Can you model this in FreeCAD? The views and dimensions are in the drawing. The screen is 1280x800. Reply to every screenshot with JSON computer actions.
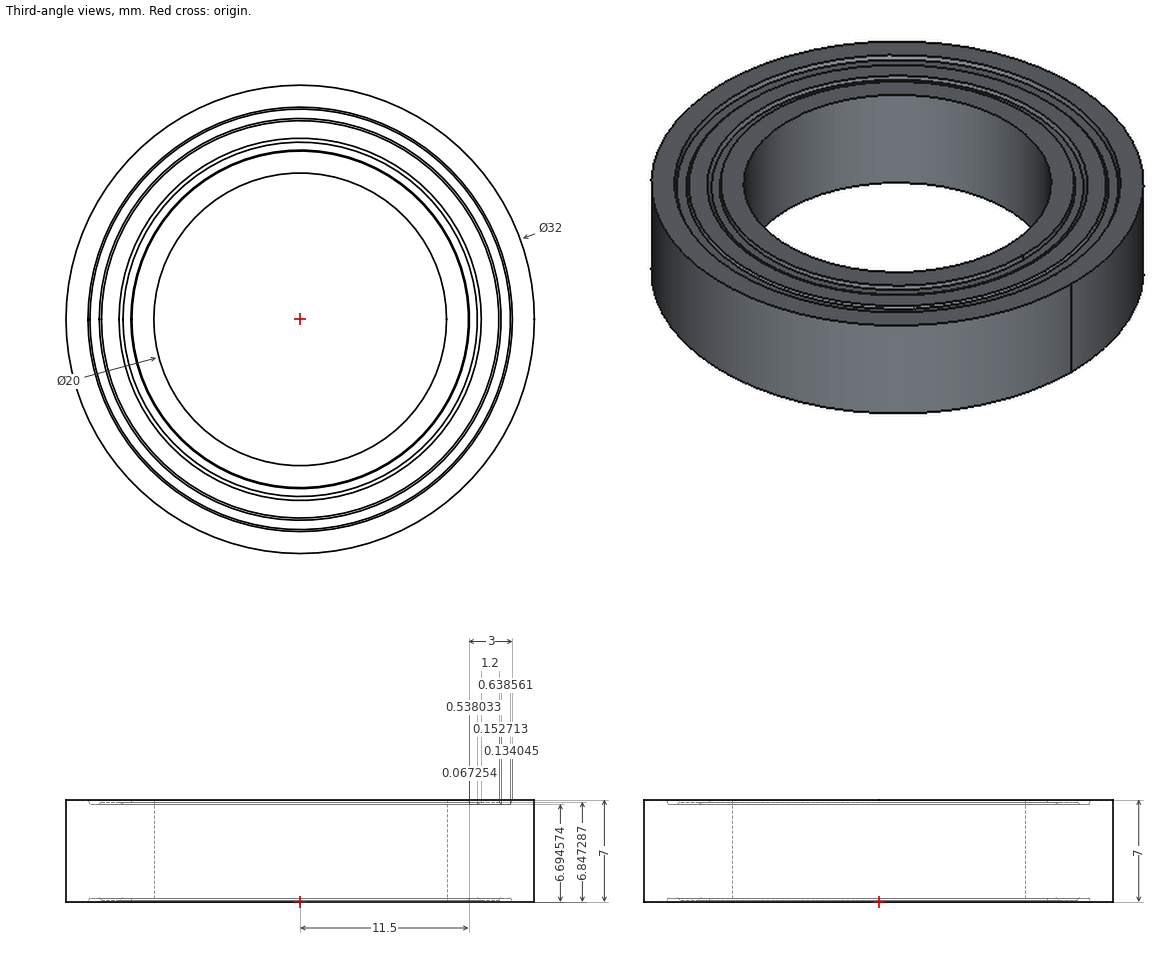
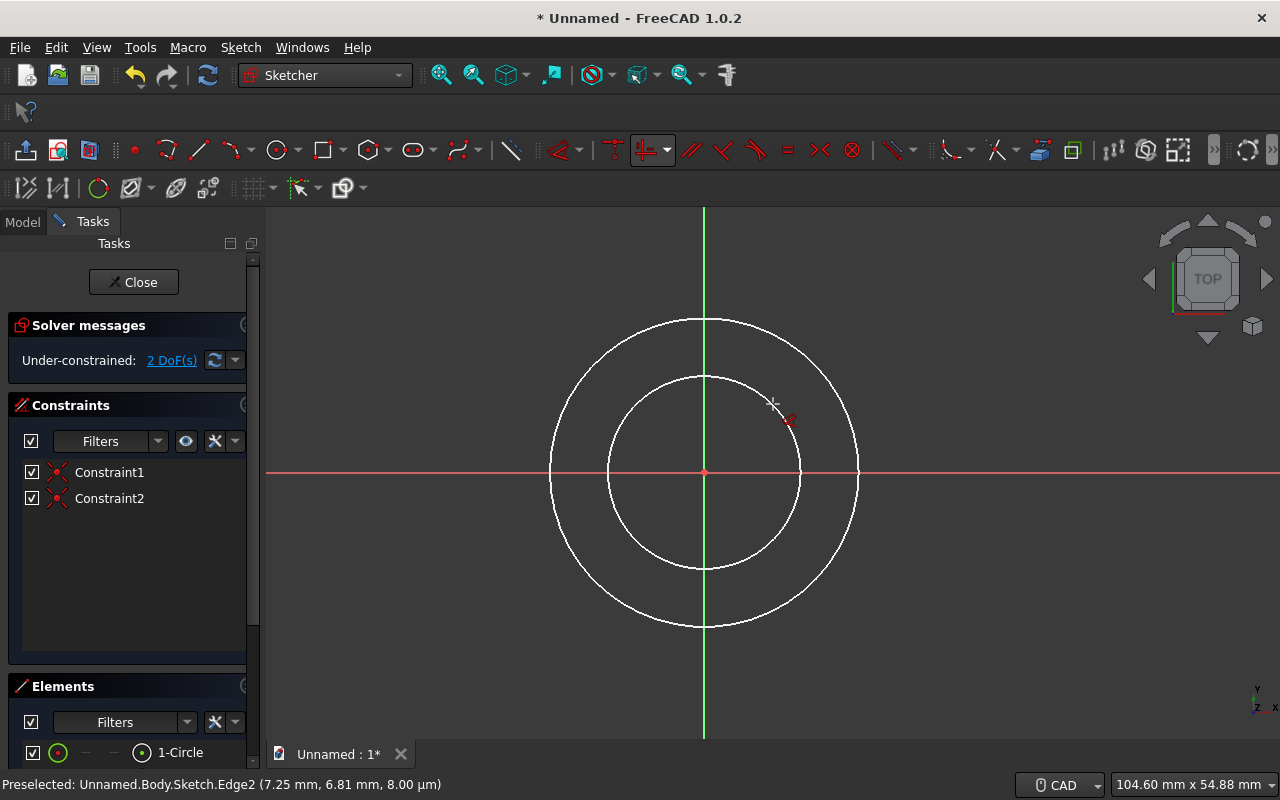
{"action": "left_click", "coordinate": [813, 363]}
{"action": "left_click", "coordinate": [836, 340]}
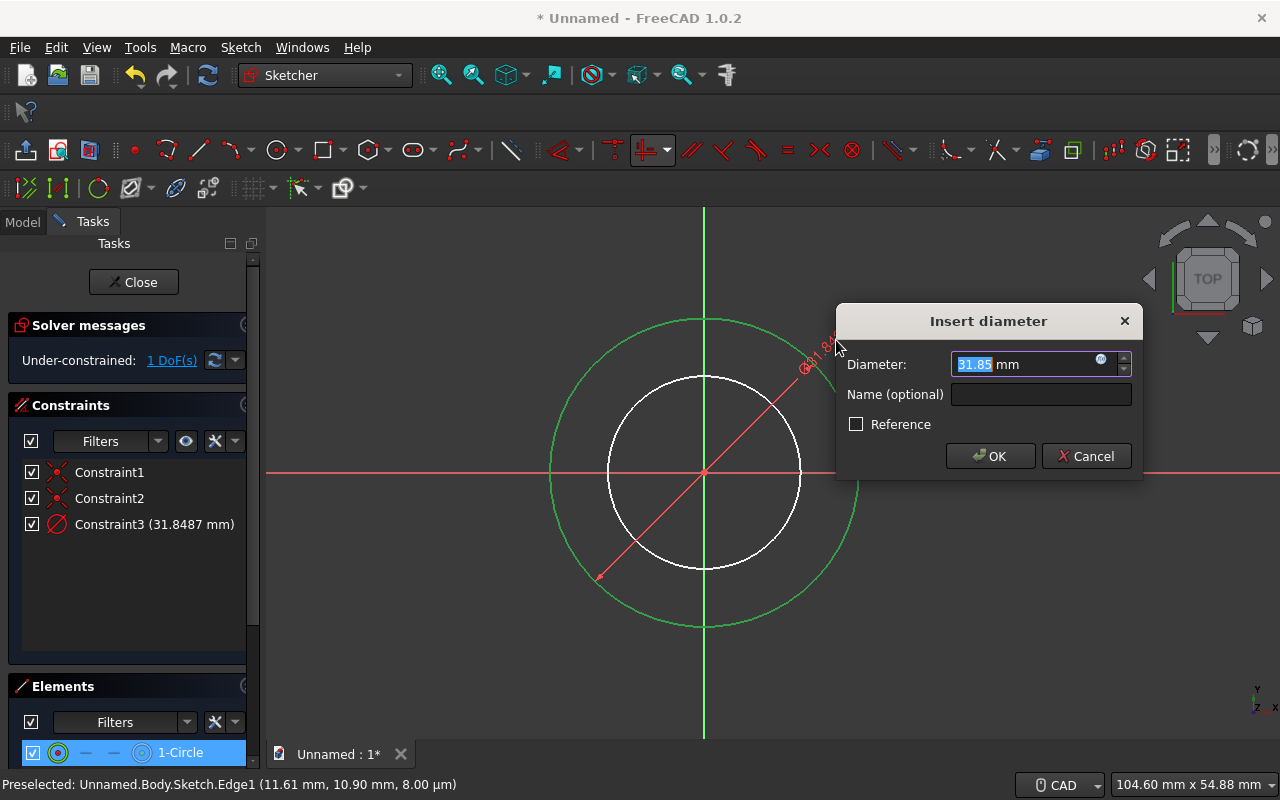
{"action": "type", "text": "32"}
{"action": "key", "text": "Return"}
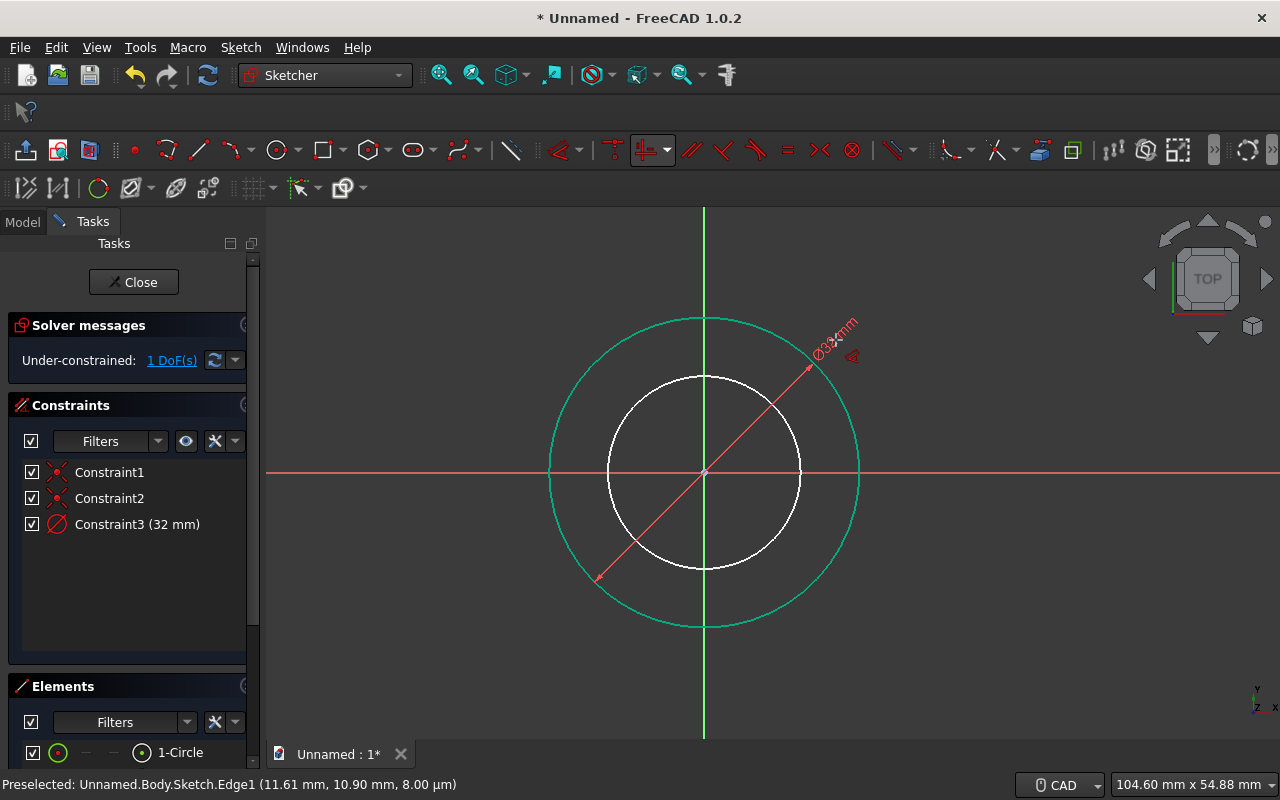
{"action": "left_click", "coordinate": [772, 404]}
{"action": "left_click", "coordinate": [794, 381]}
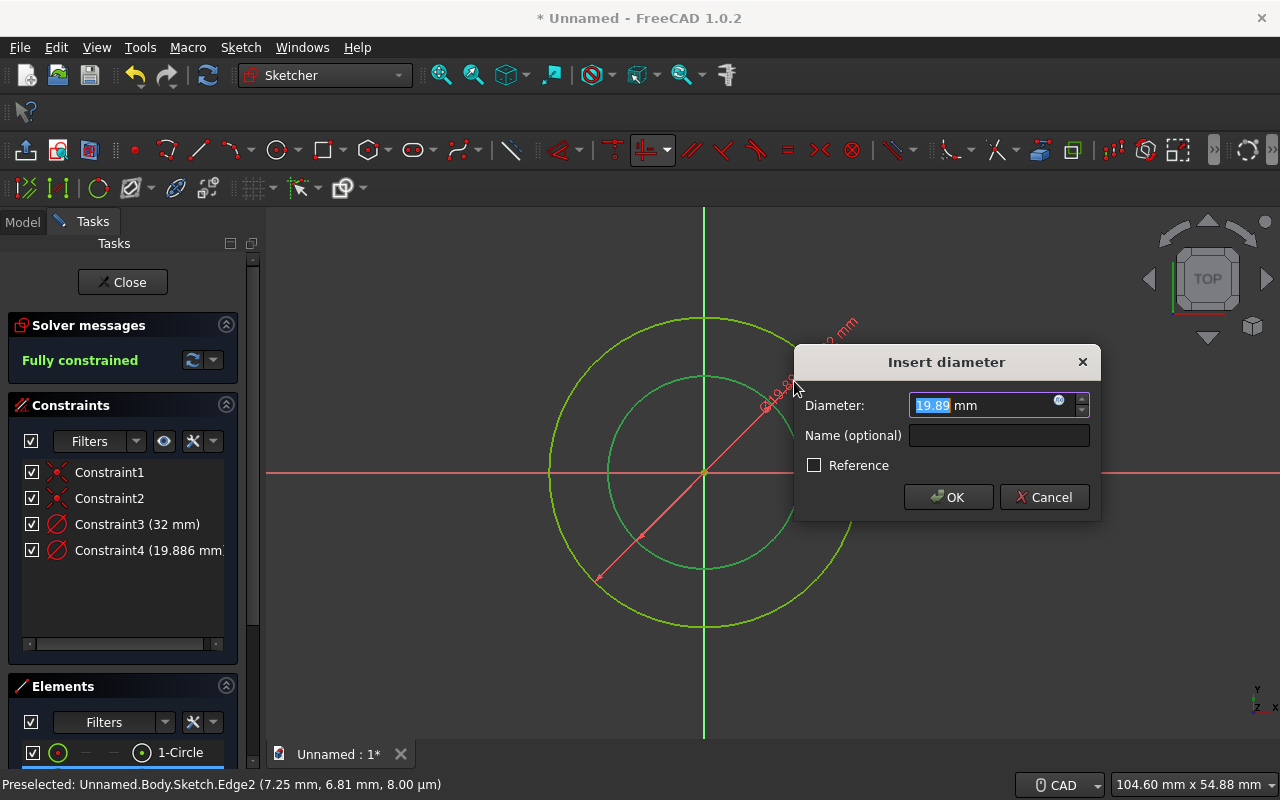
{"action": "type", "text": "20"}
{"action": "key", "text": "Return"}
{"action": "key", "text": "Escape"}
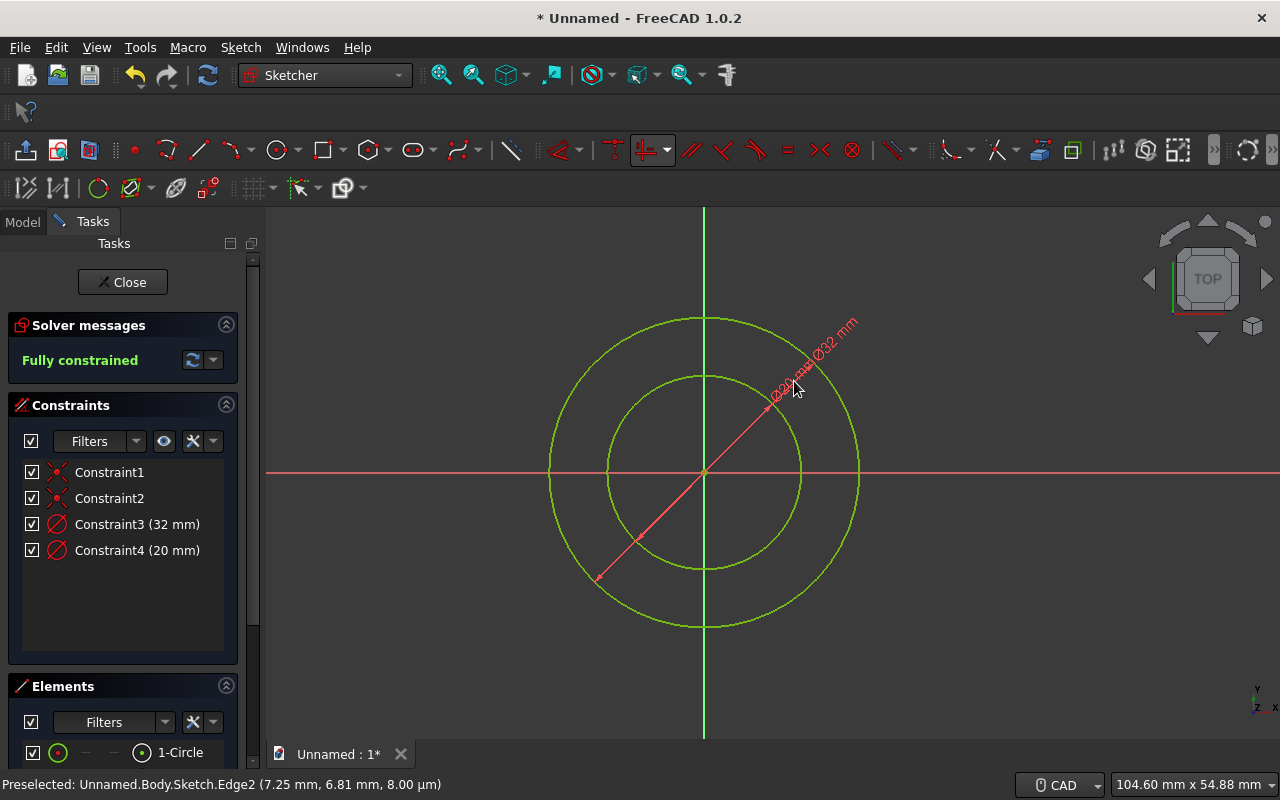
{"action": "left_click", "coordinate": [123, 282]}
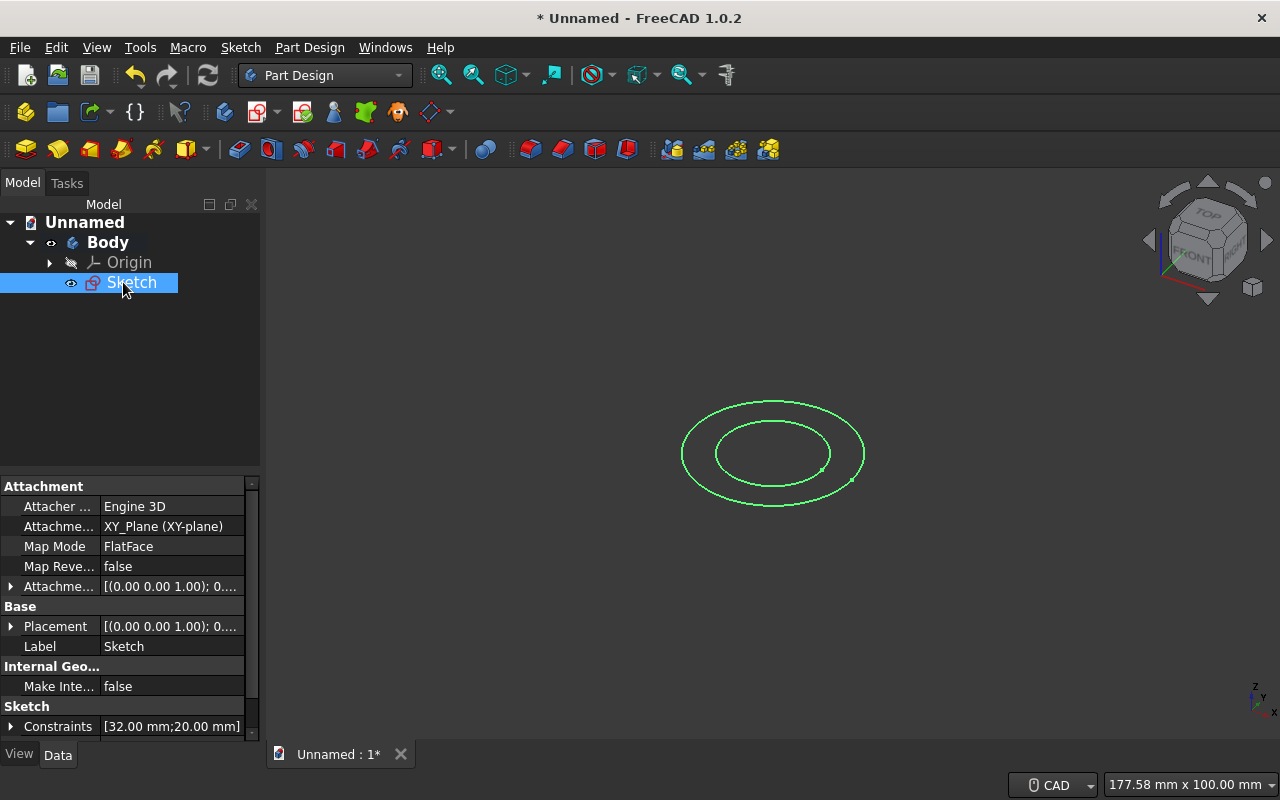
{"action": "left_click", "coordinate": [26, 150]}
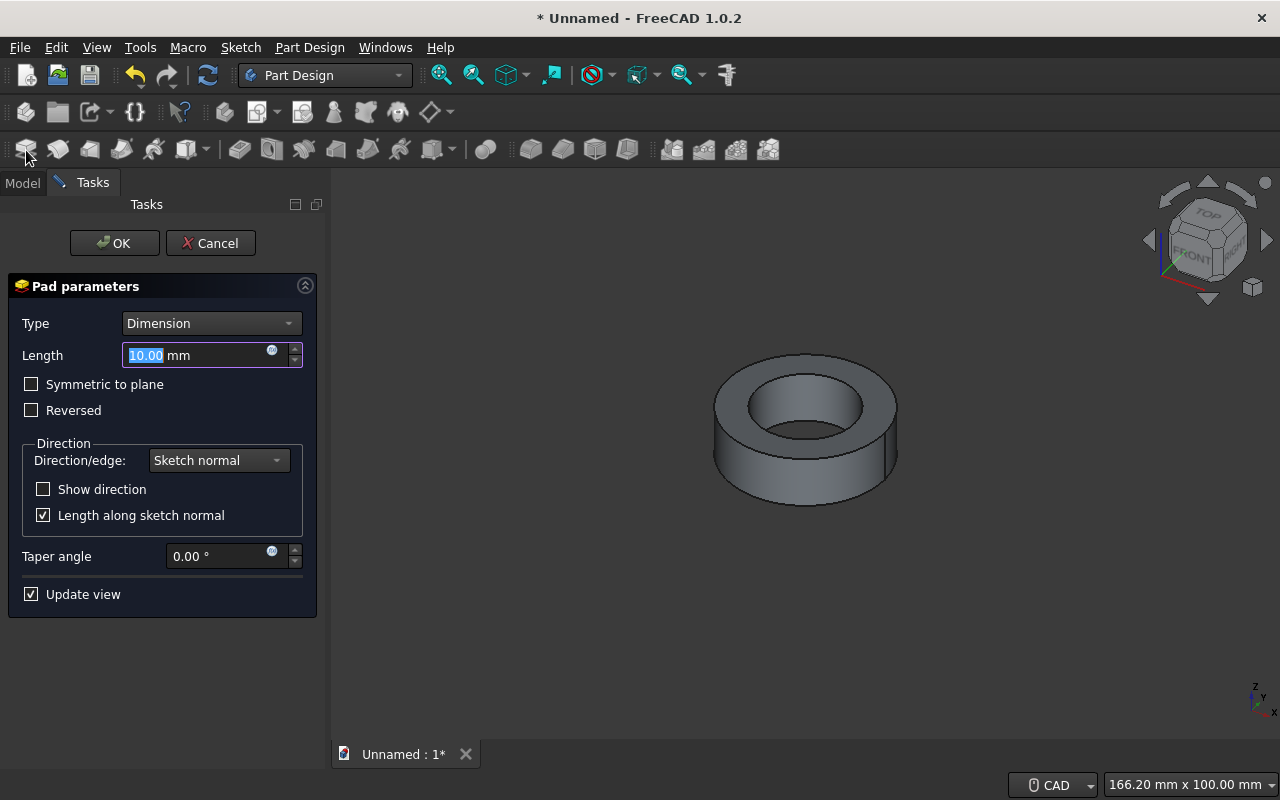
{"action": "type", "text": "7"}
{"action": "key", "text": "Tab"}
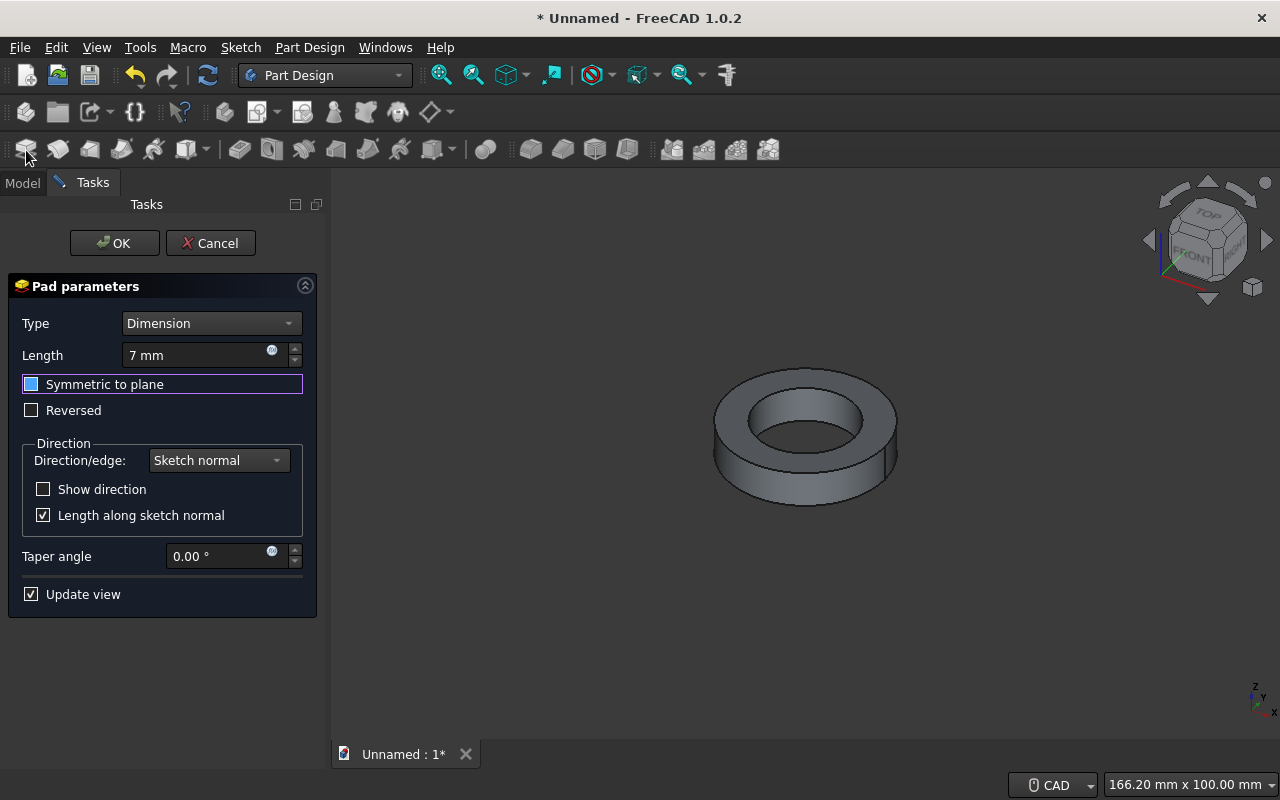
{"action": "left_click", "coordinate": [115, 243]}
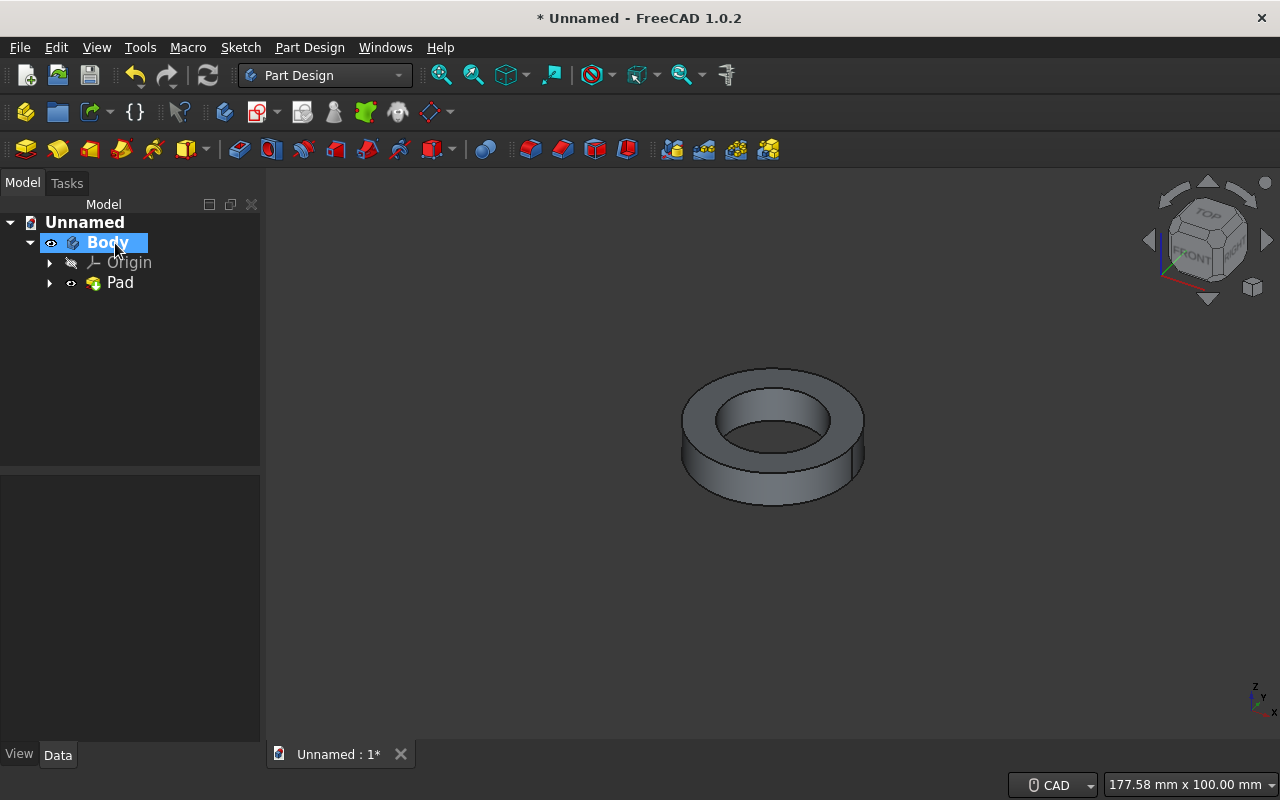
{"action": "key", "text": "v f"}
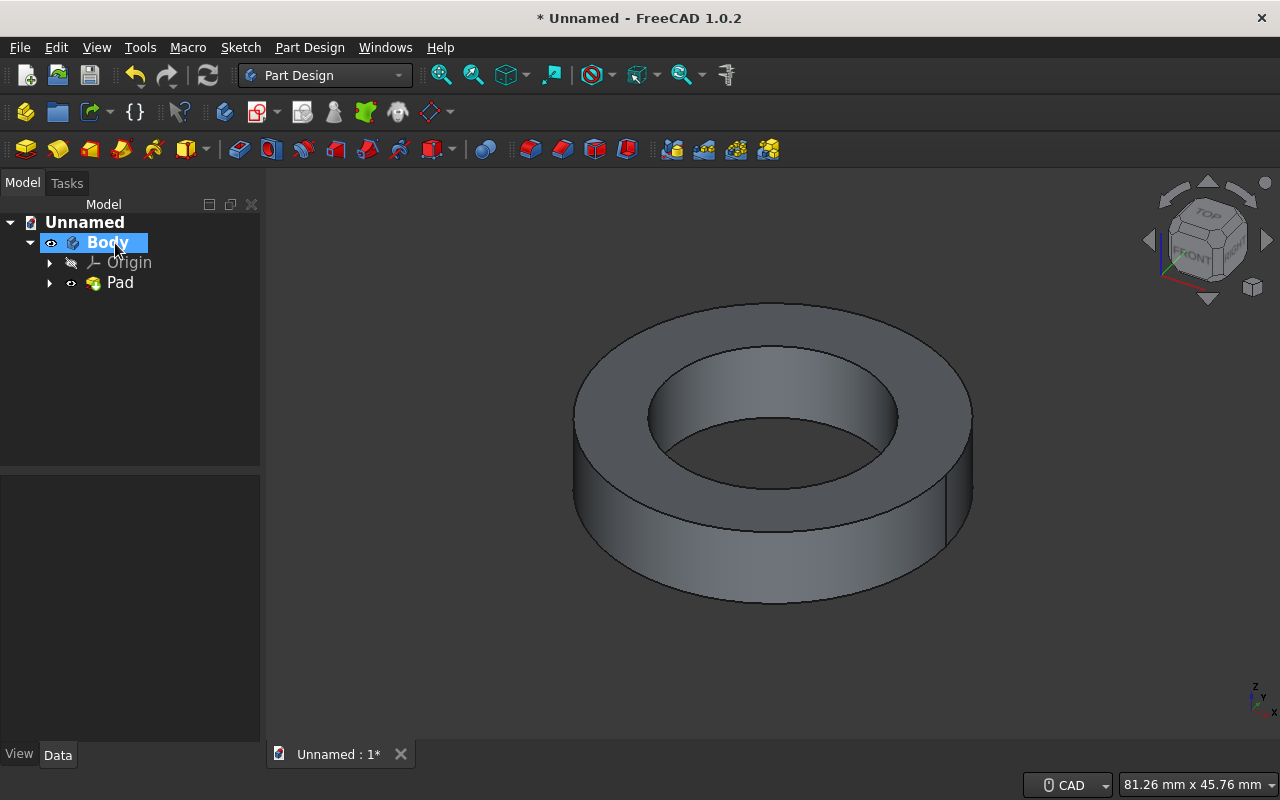
{"action": "left_click", "coordinate": [258, 112]}